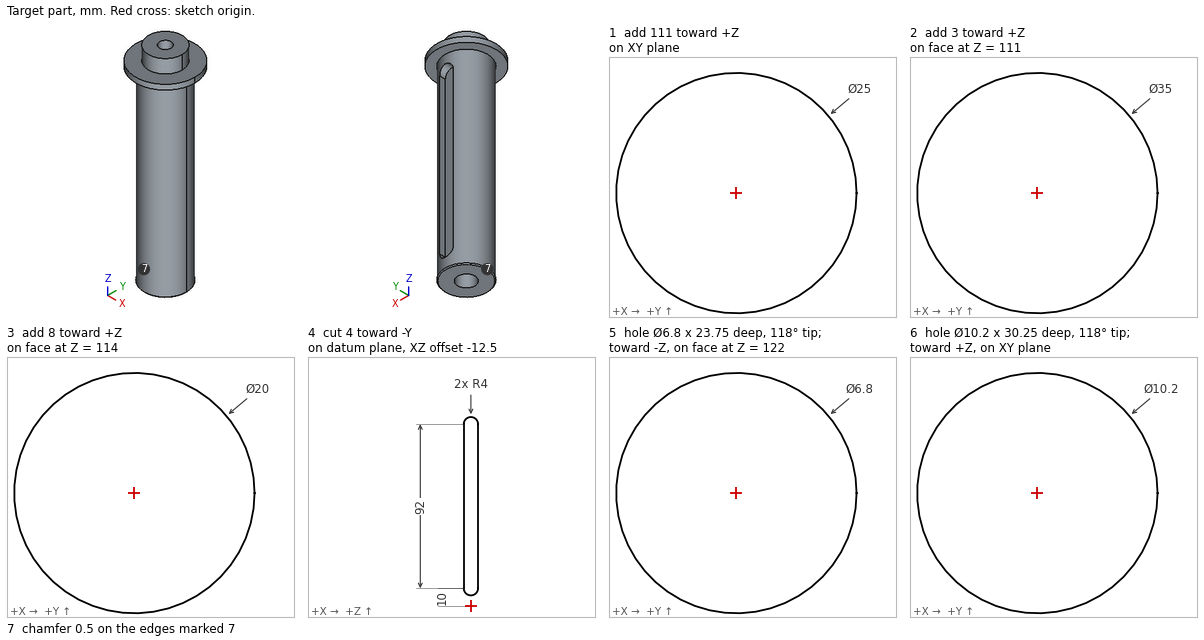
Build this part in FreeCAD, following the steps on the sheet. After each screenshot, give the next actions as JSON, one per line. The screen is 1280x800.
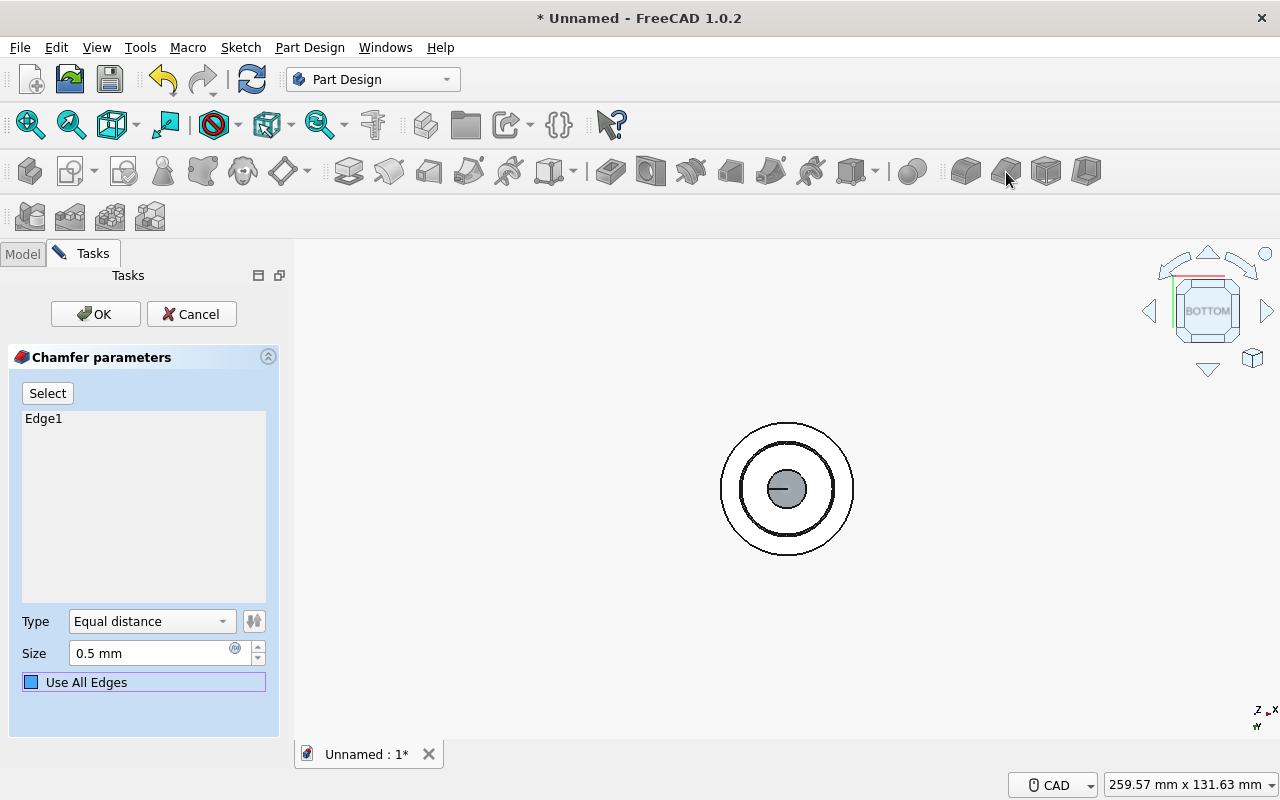
{"action": "left_click", "coordinate": [96, 314]}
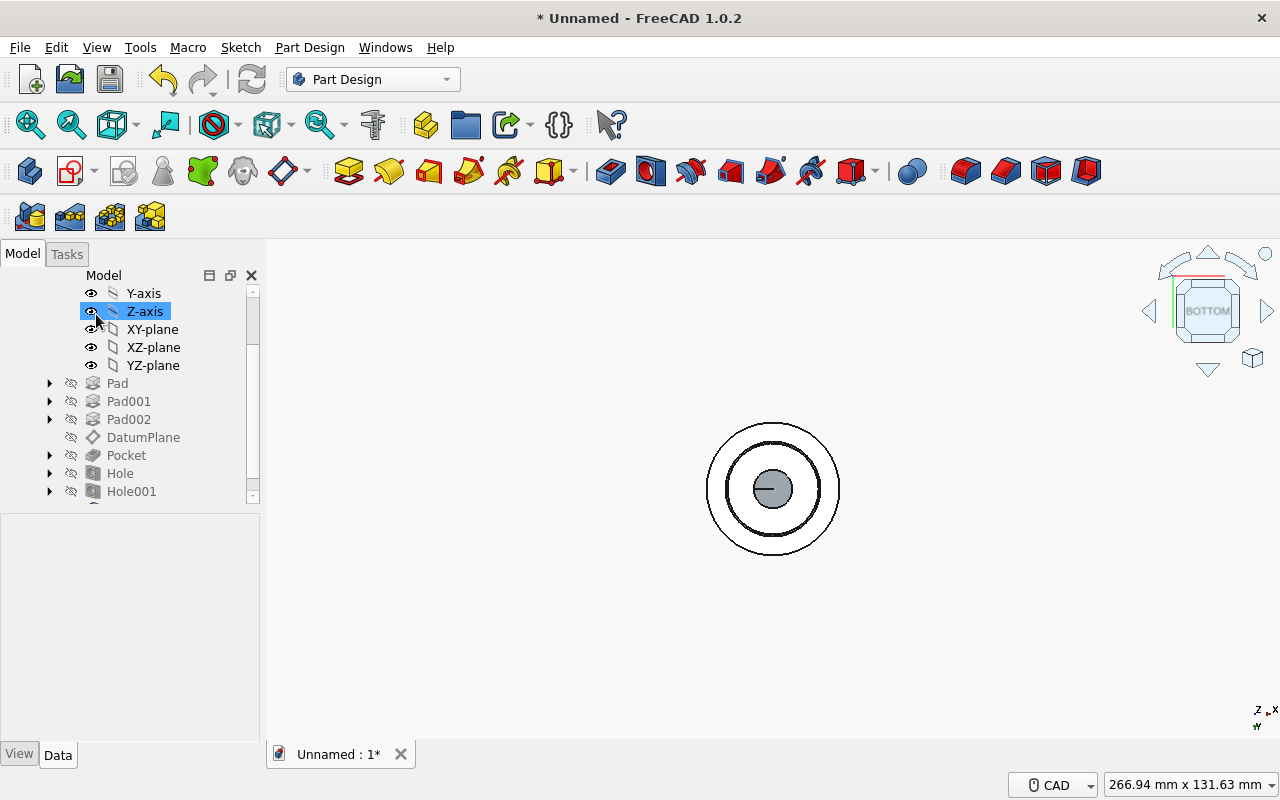
{"action": "key", "text": "0"}